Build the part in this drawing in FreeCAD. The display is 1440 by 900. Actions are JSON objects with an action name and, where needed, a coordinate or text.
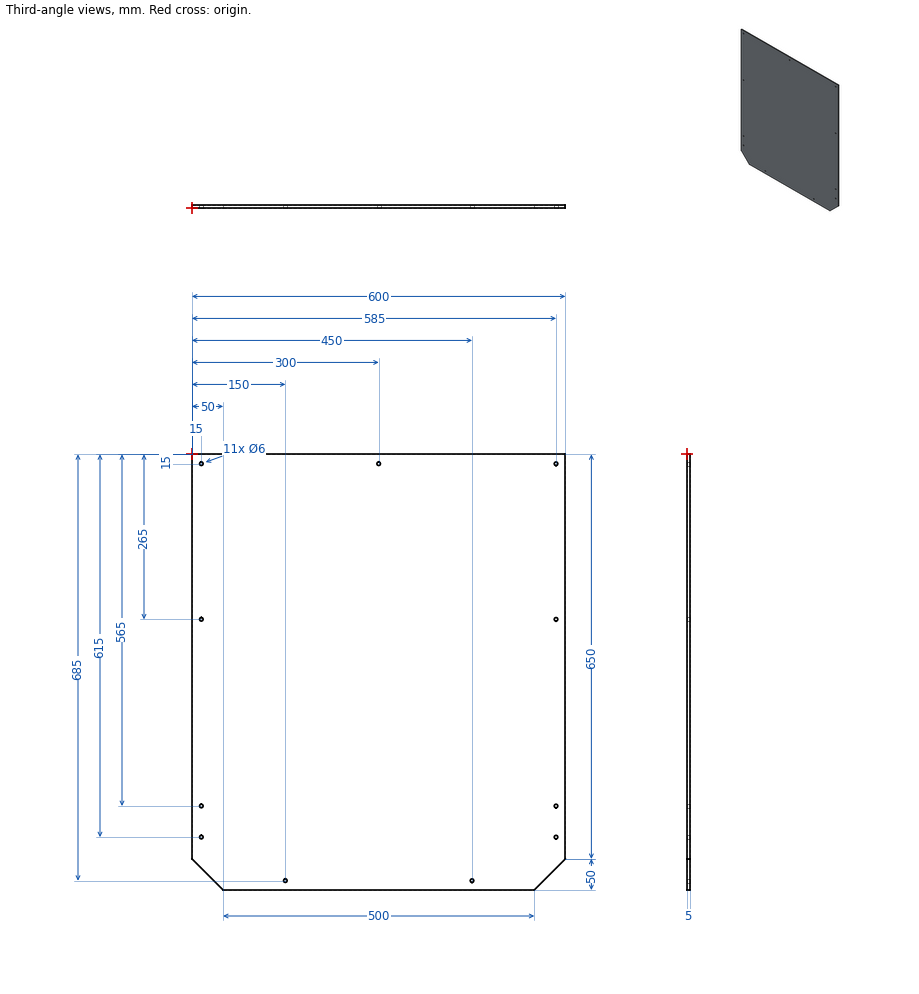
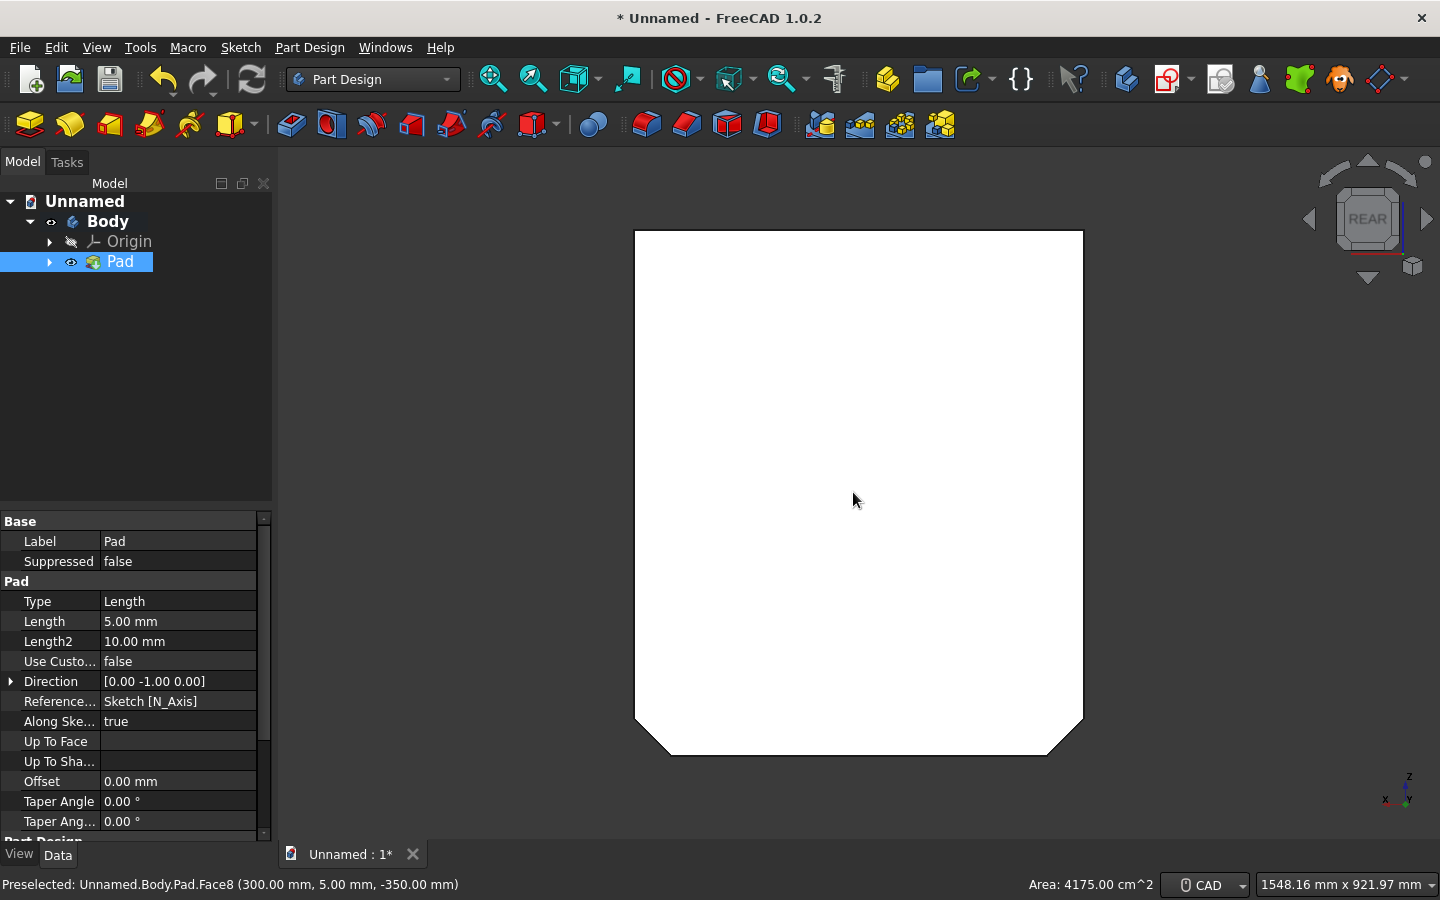
{"action": "left_click", "coordinate": [1168, 80]}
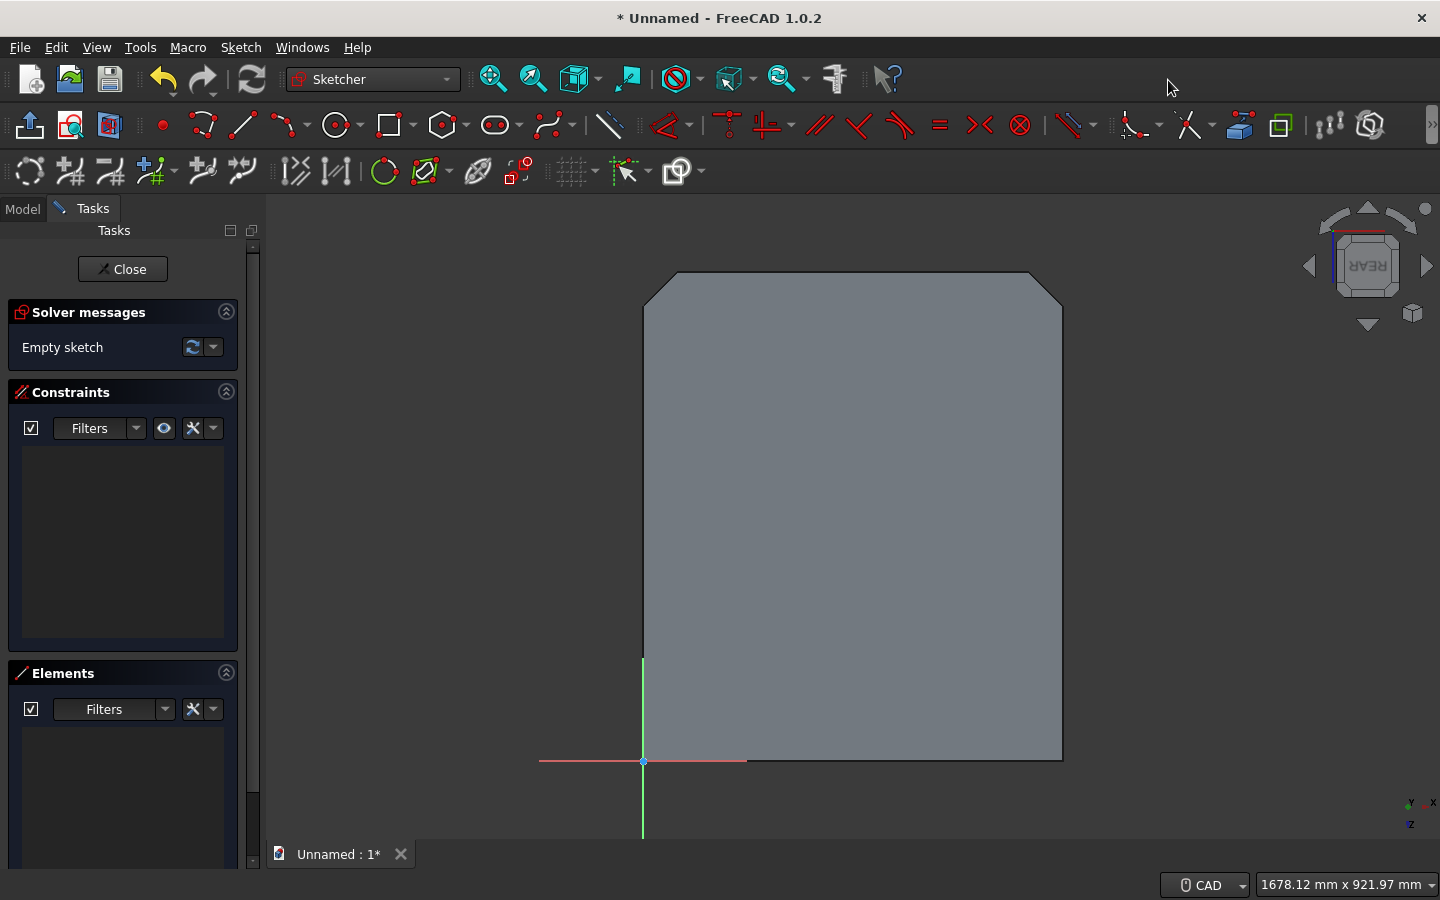
{"action": "key", "text": "g c"}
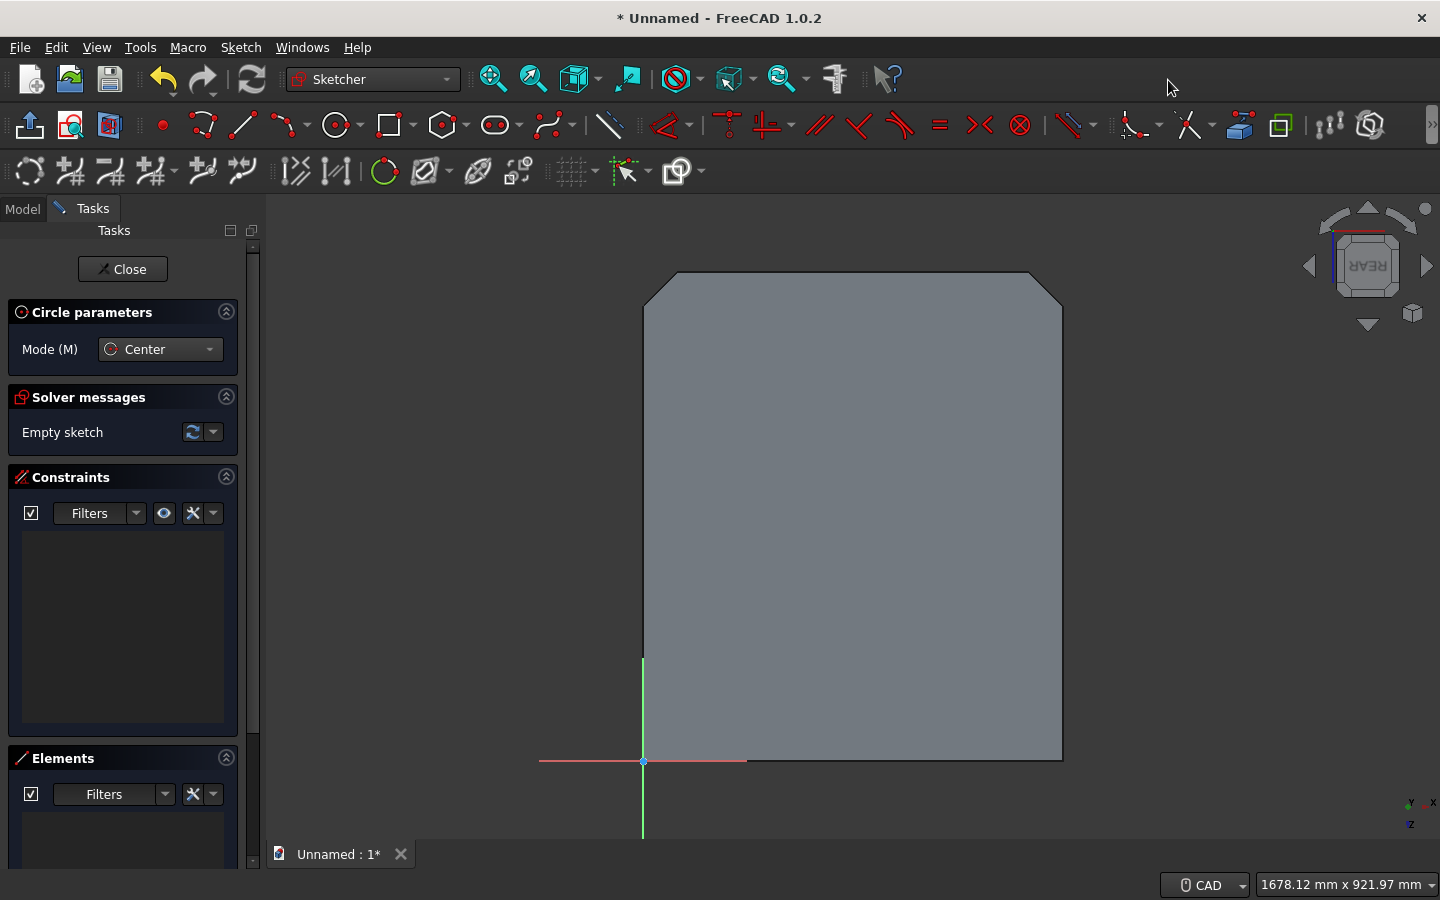
{"action": "scroll", "coordinate": [654, 751], "scroll_direction": "up", "scroll_amount": 12}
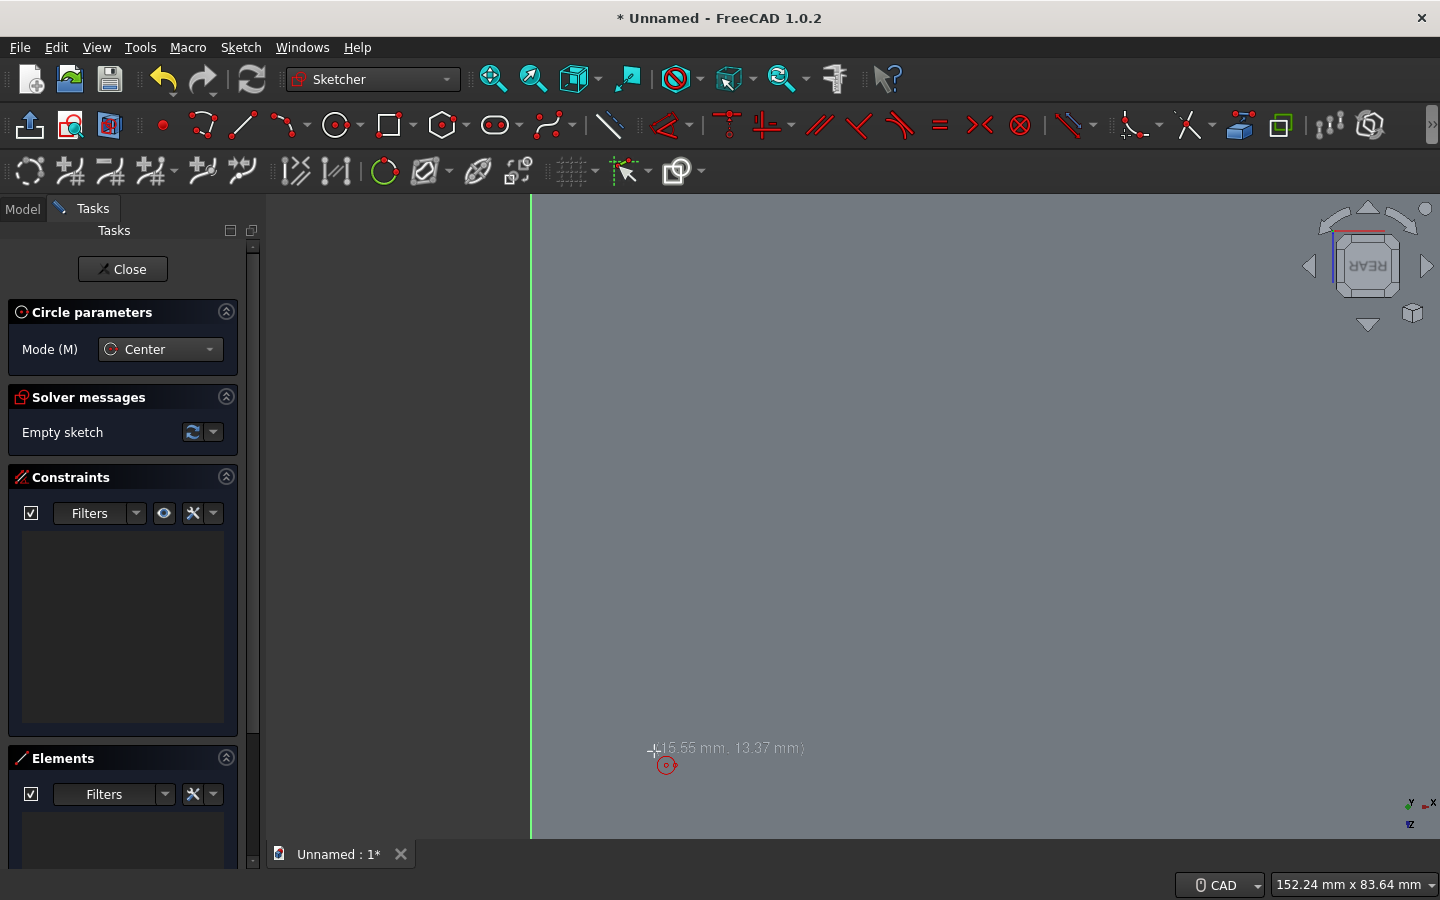
{"action": "scroll", "coordinate": [623, 702], "scroll_direction": "down", "scroll_amount": 13}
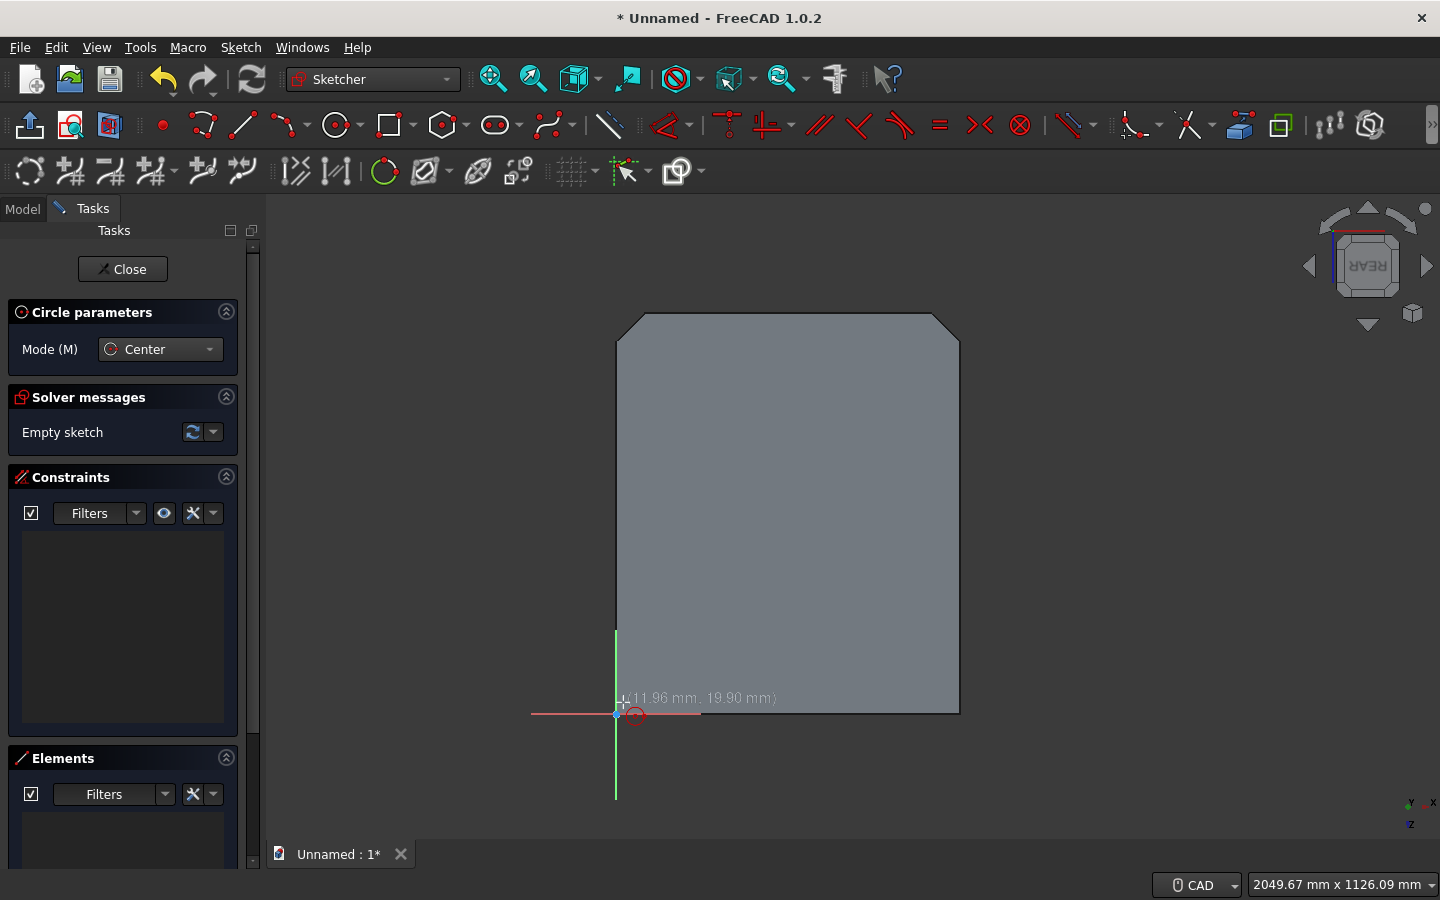
{"action": "scroll", "coordinate": [625, 706], "scroll_direction": "up", "scroll_amount": 4}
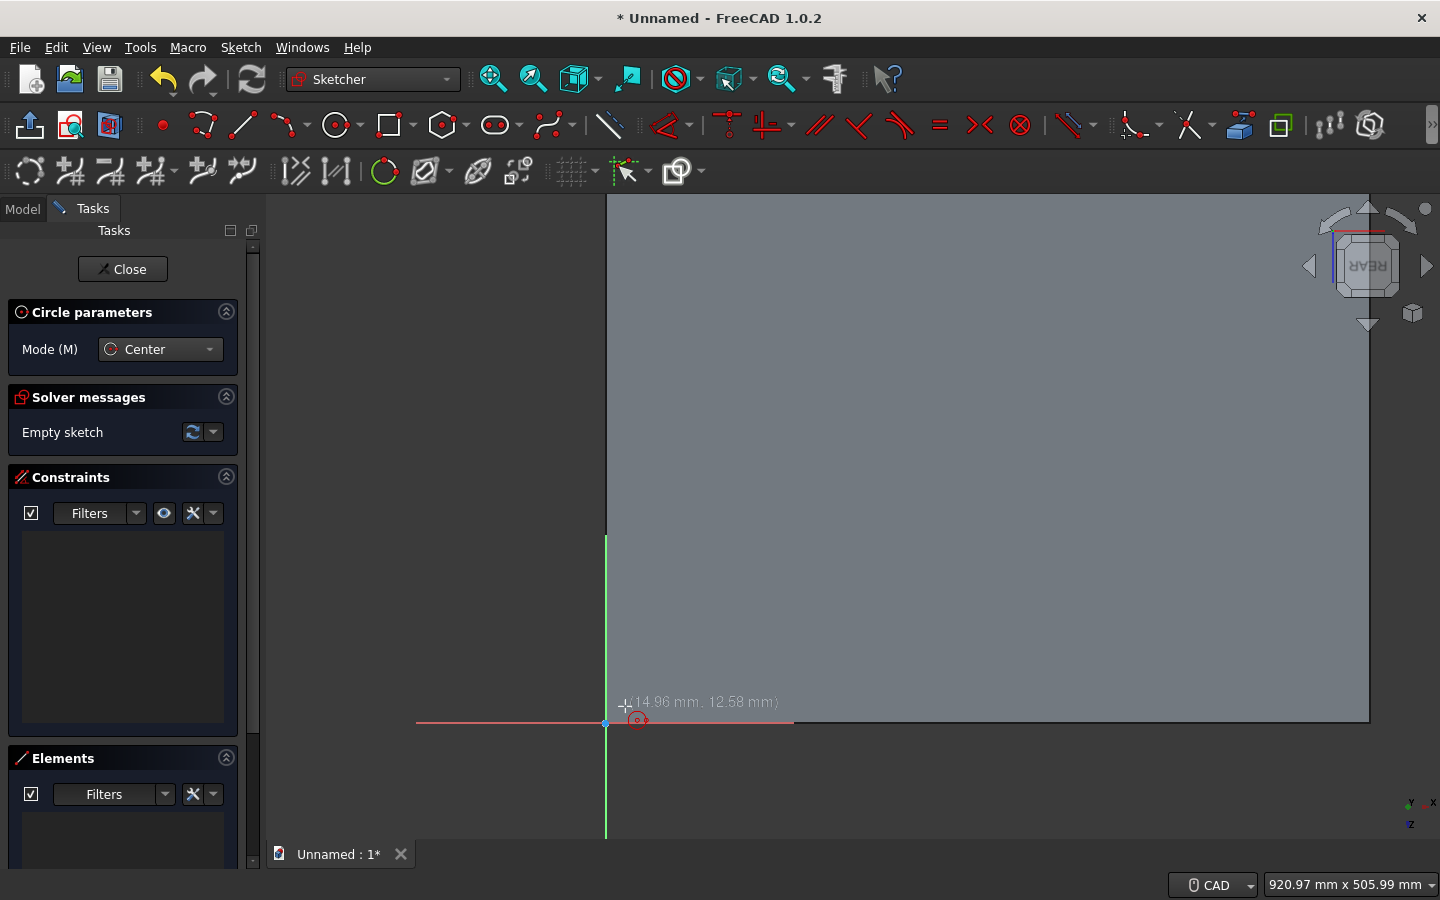
{"action": "left_click", "coordinate": [625, 704]}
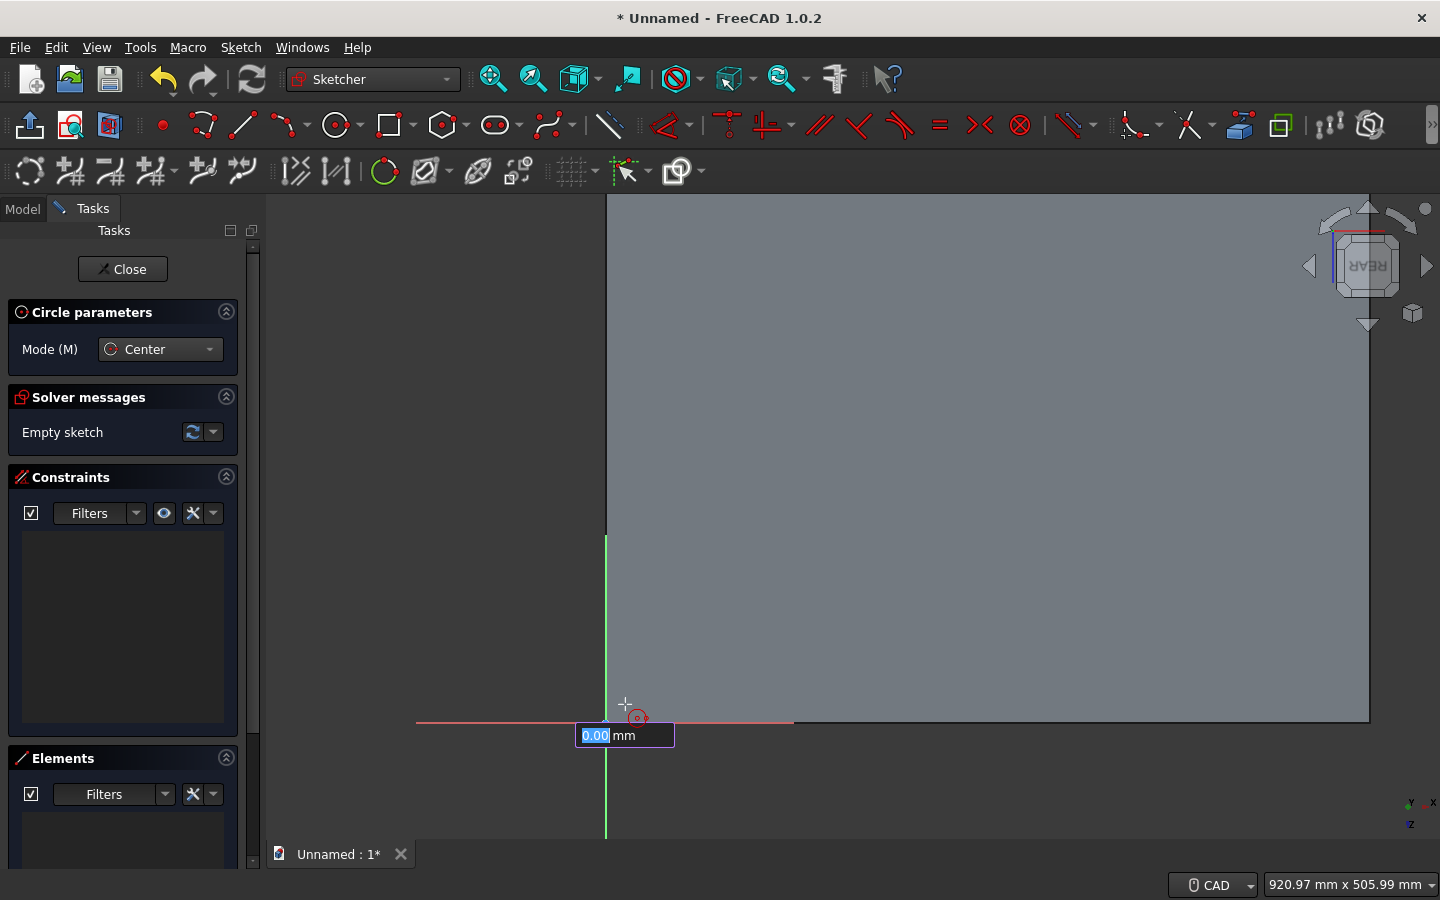
{"action": "scroll", "coordinate": [627, 701], "scroll_direction": "up", "scroll_amount": 8}